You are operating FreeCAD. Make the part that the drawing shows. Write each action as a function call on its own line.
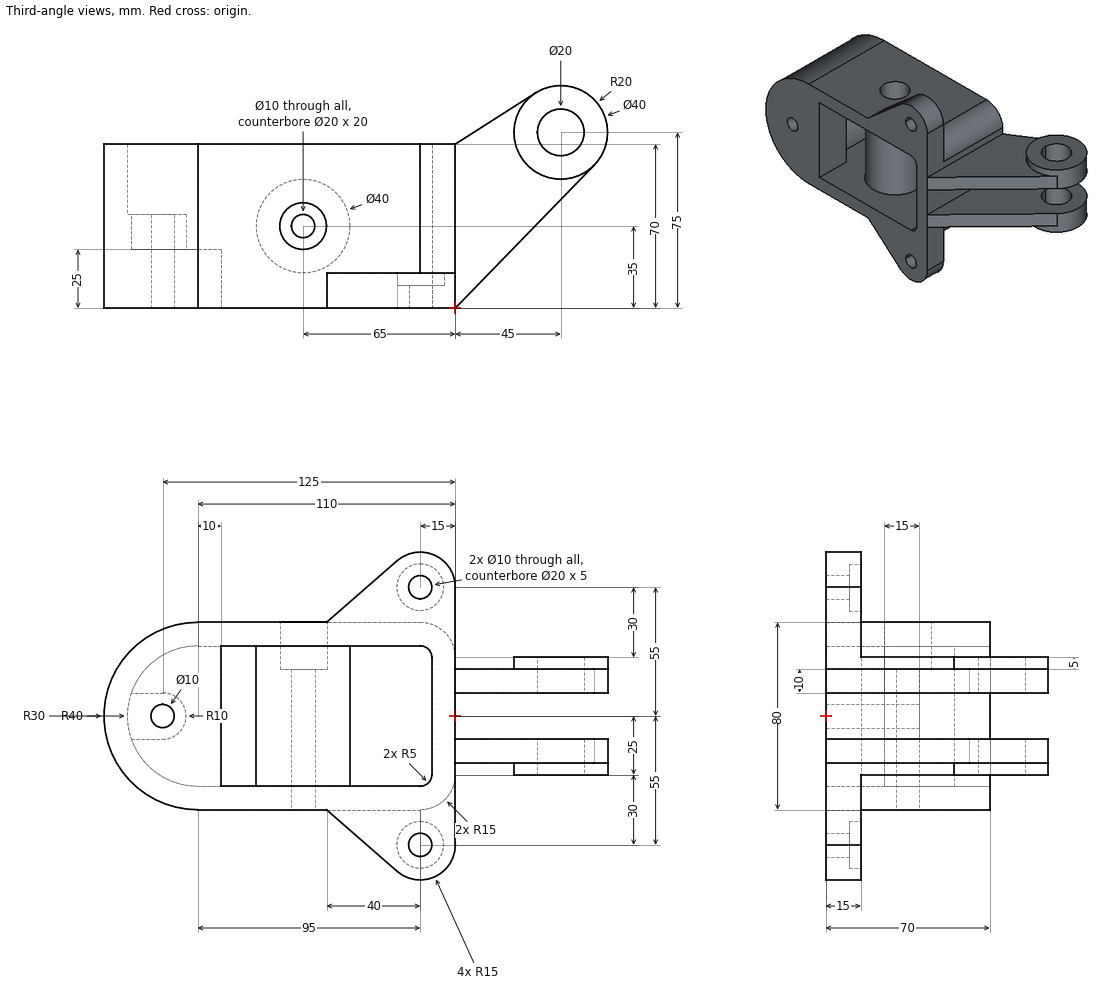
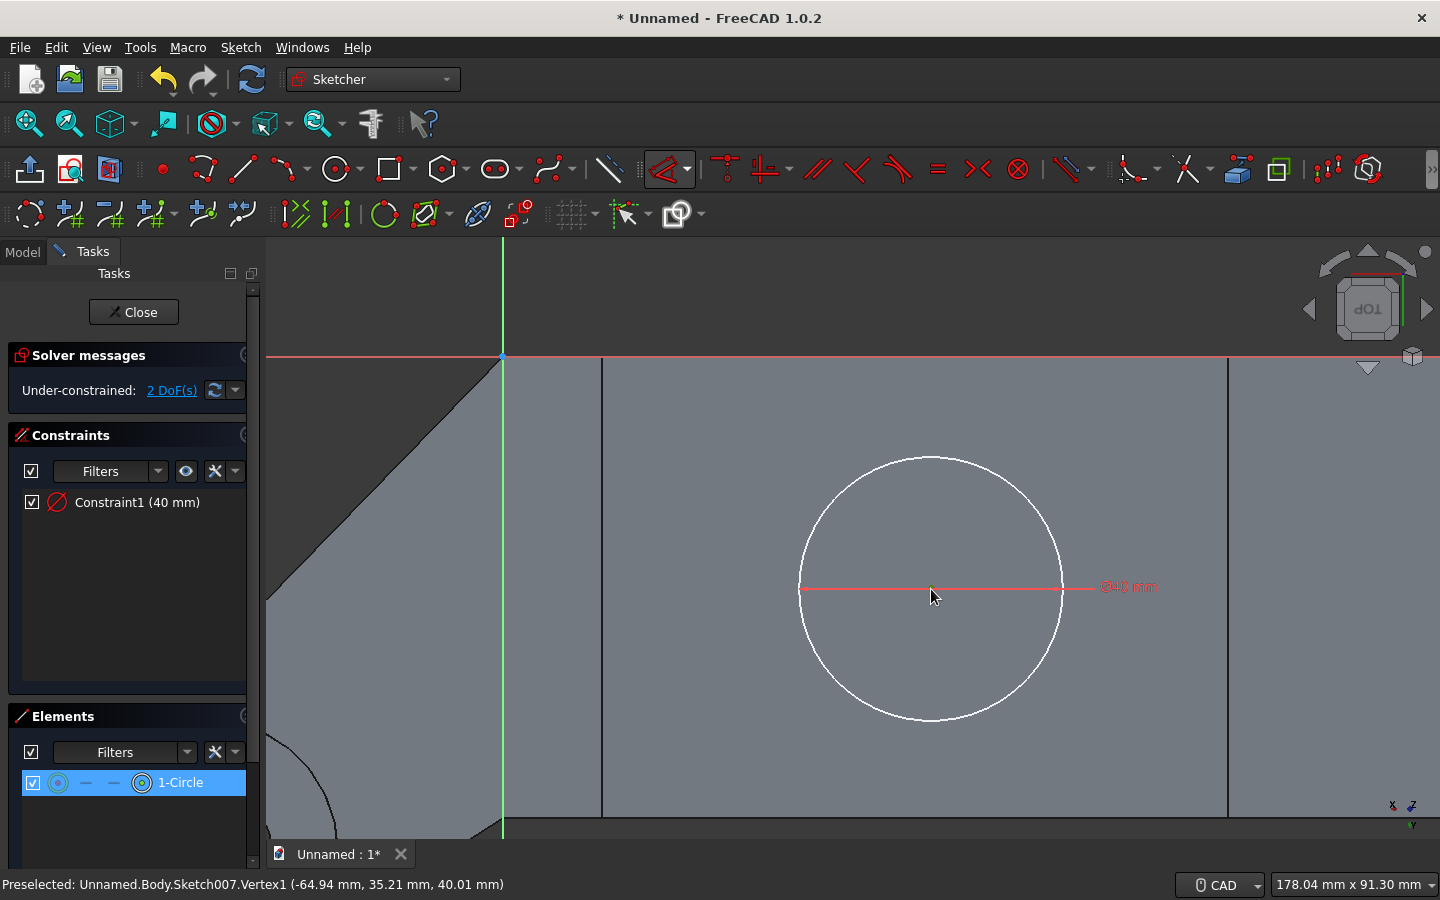
key(l)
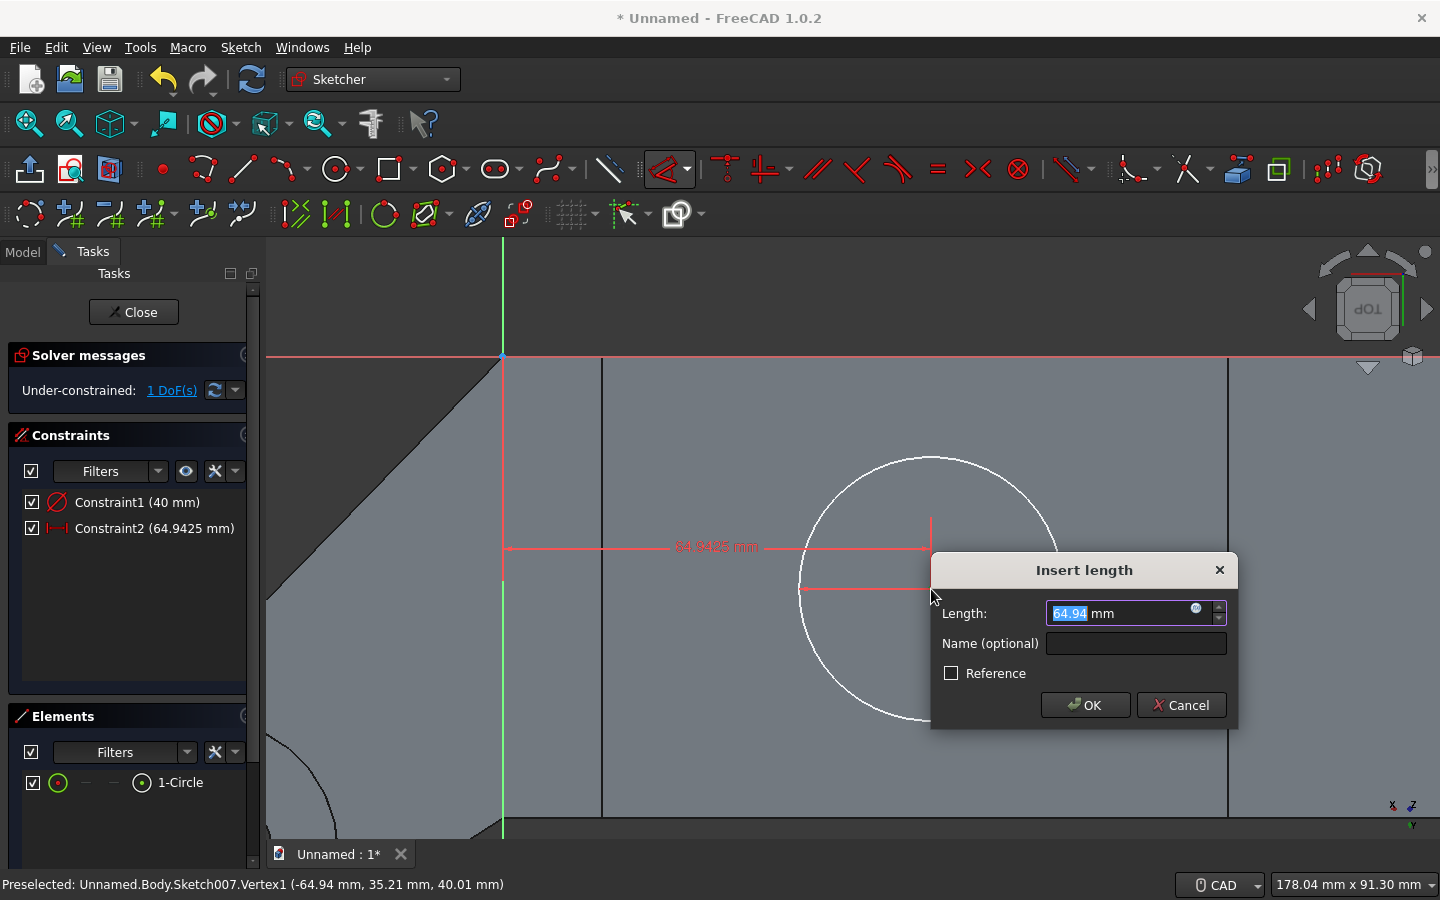
text(65)
key(Return)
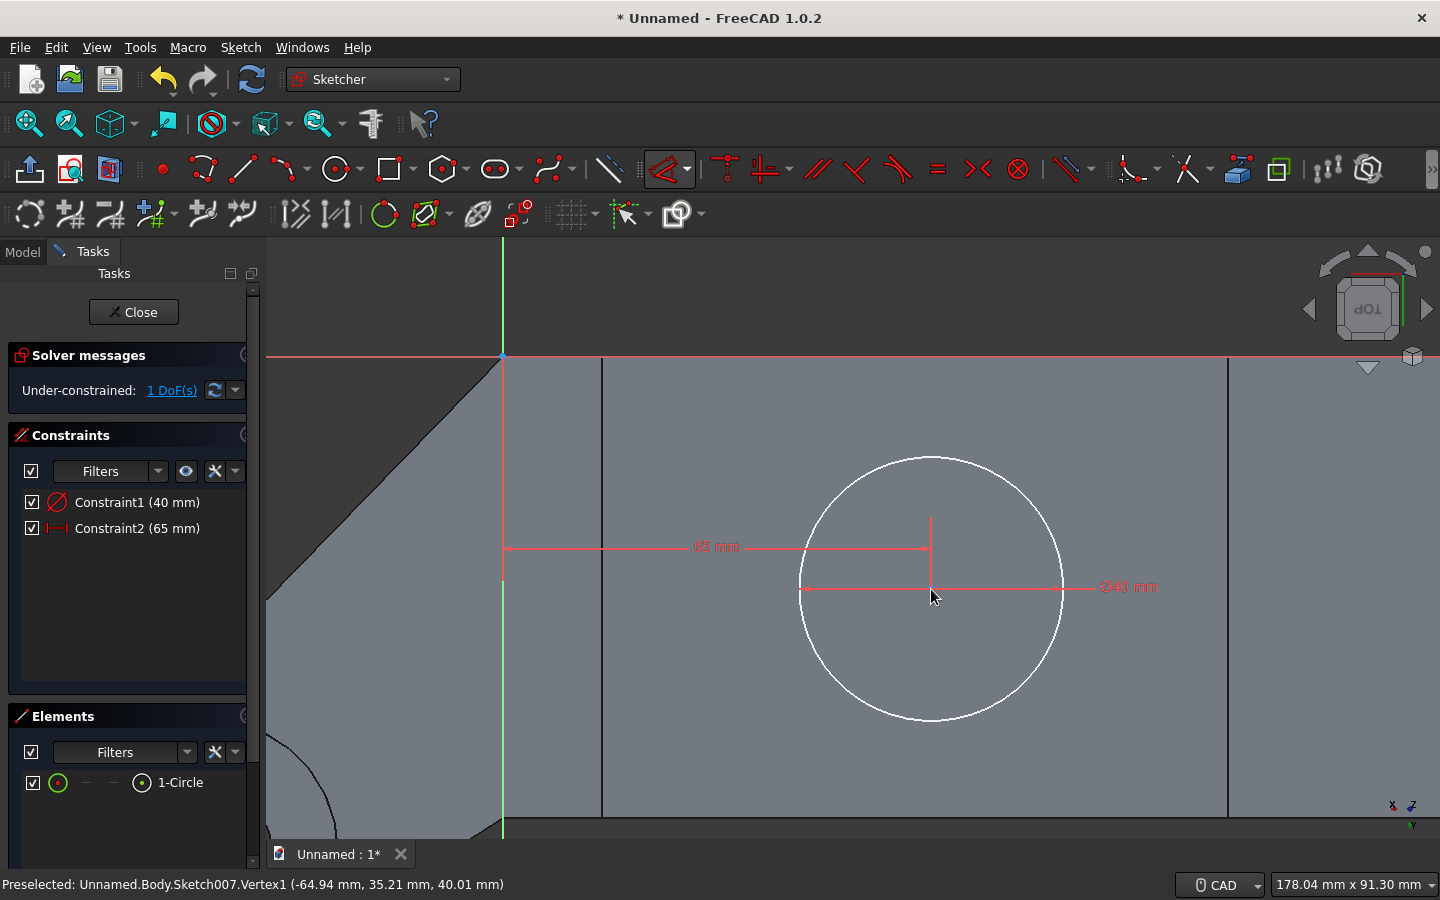
click(931, 589)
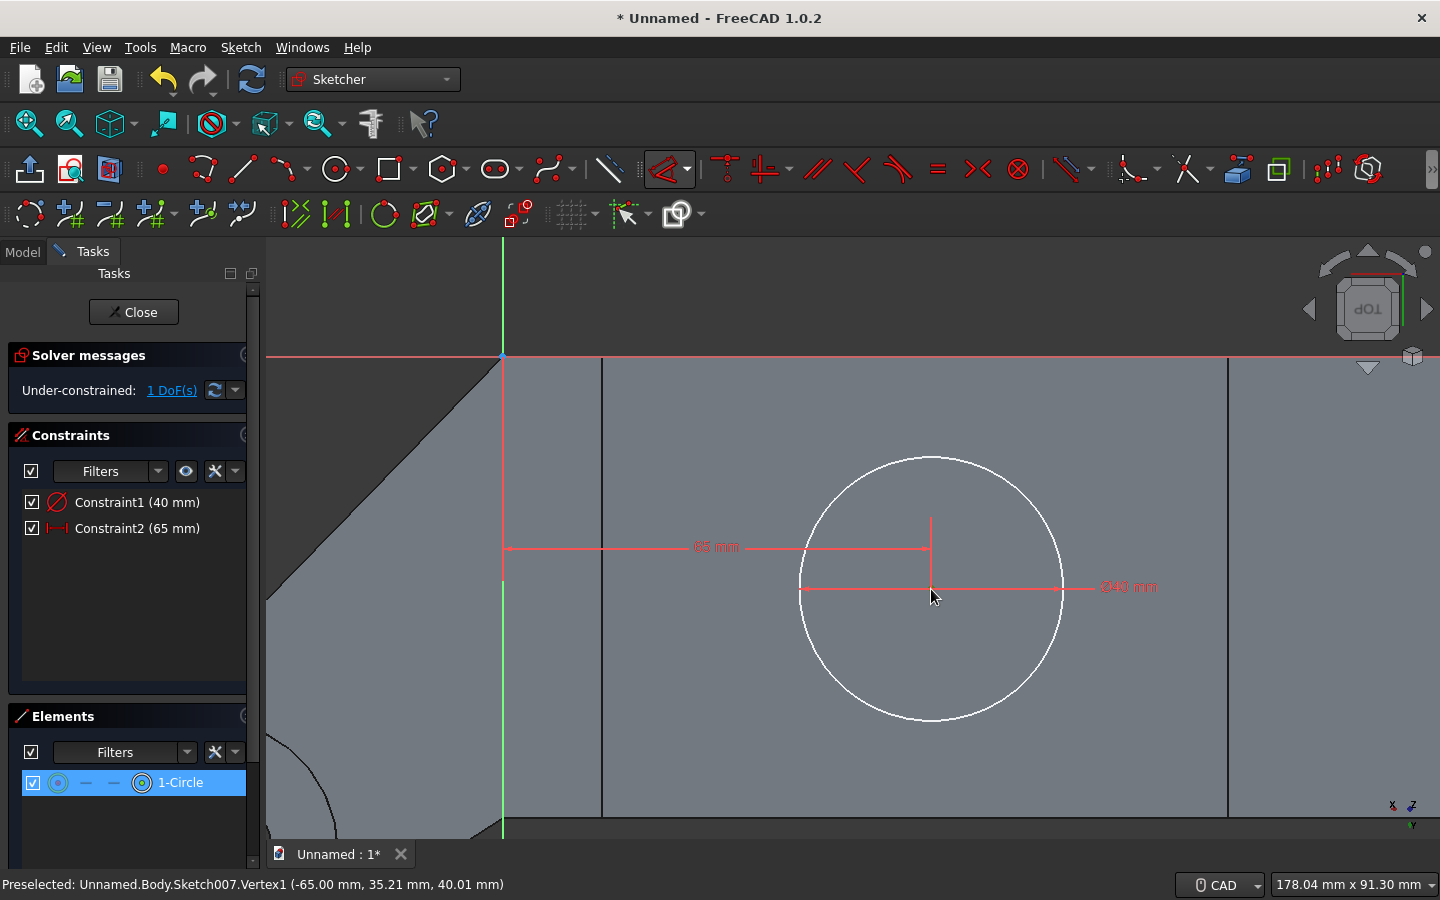
key(i)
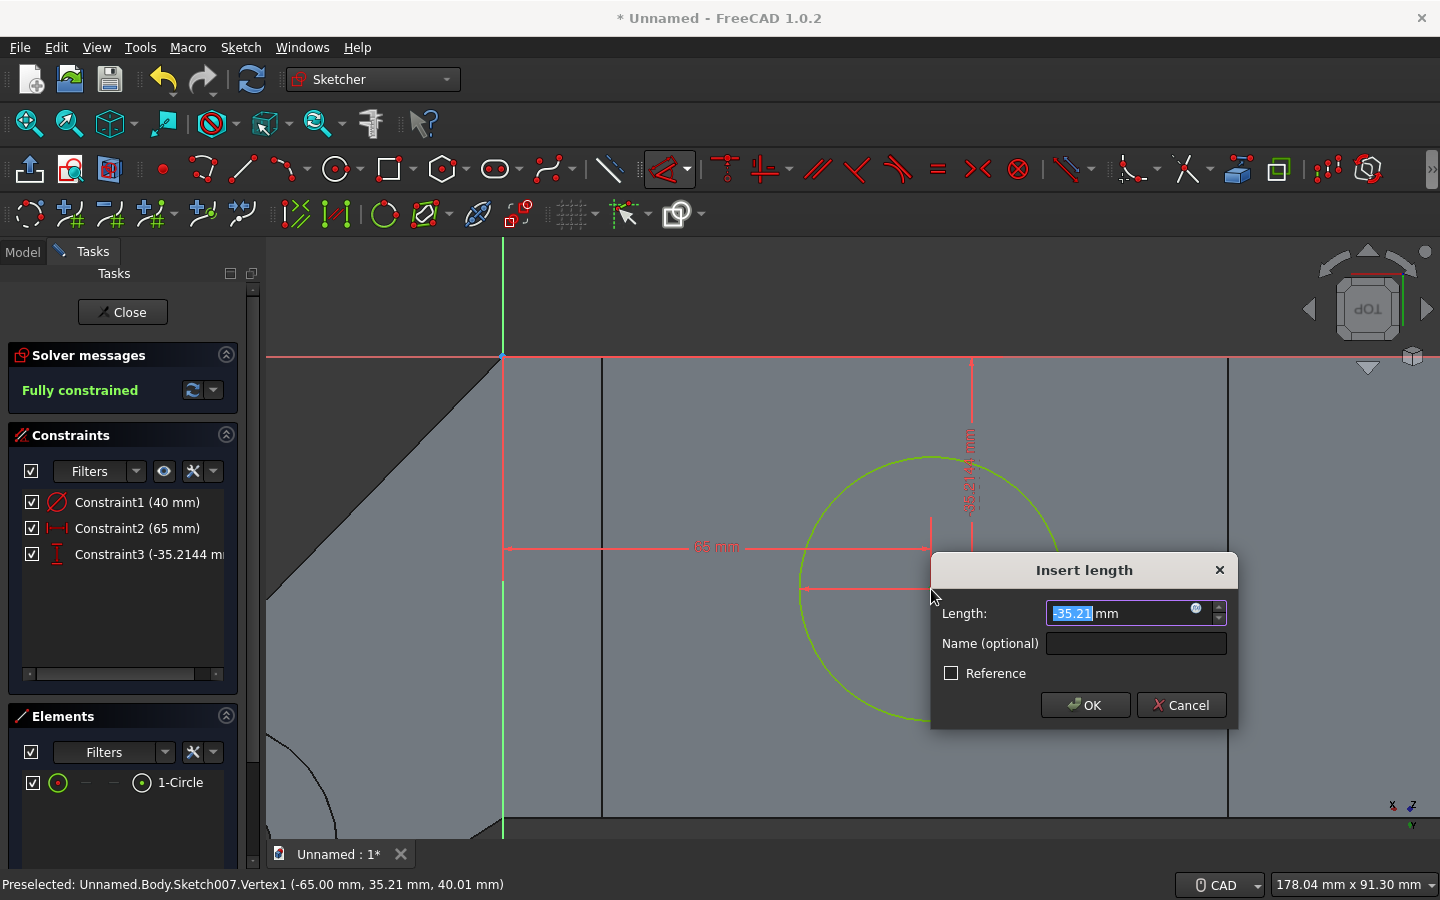
text(-35)
key(Return)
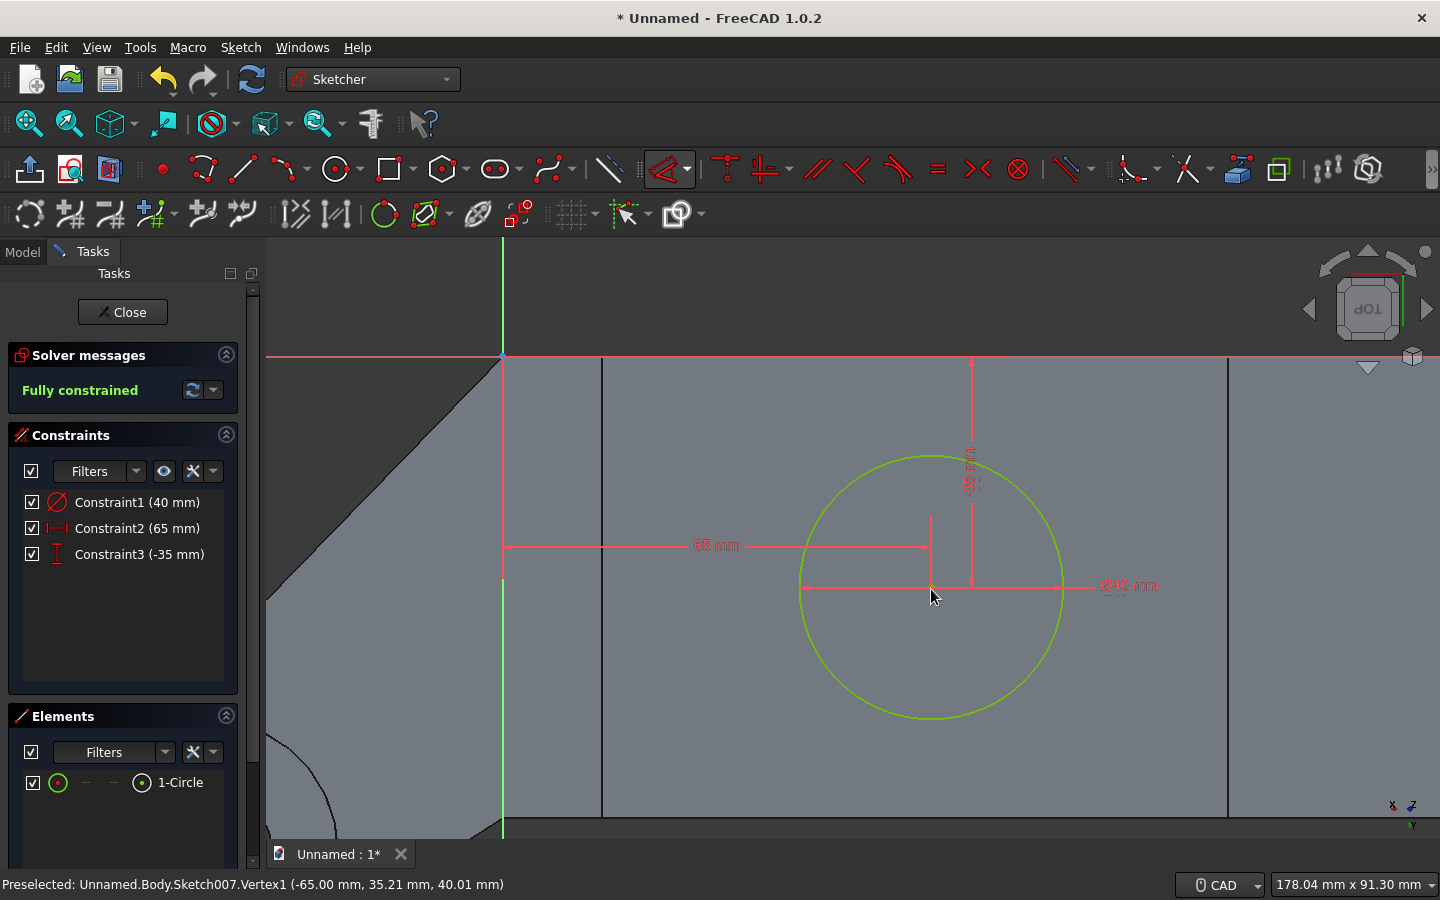
click(123, 312)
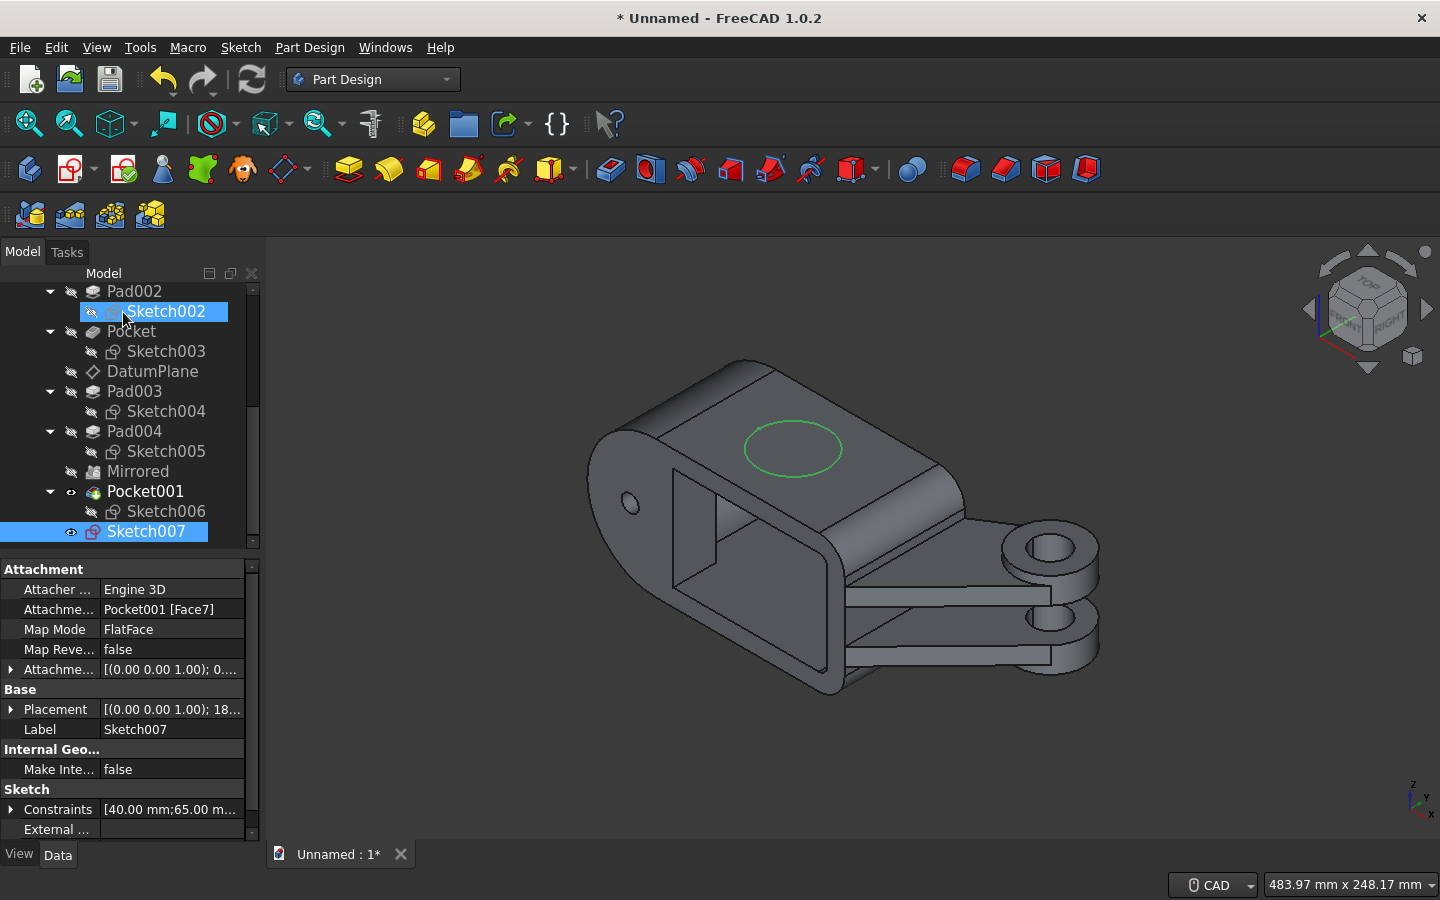
click(350, 170)